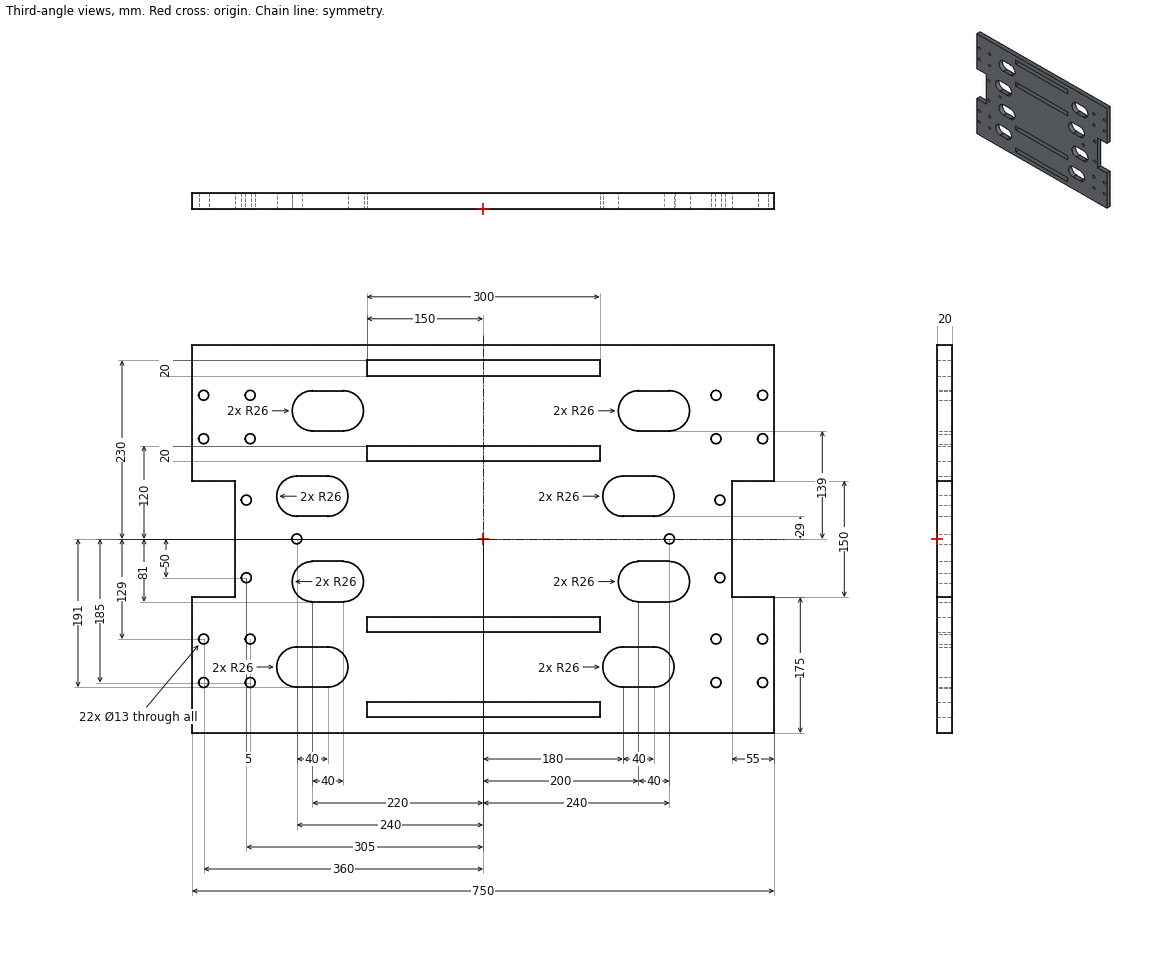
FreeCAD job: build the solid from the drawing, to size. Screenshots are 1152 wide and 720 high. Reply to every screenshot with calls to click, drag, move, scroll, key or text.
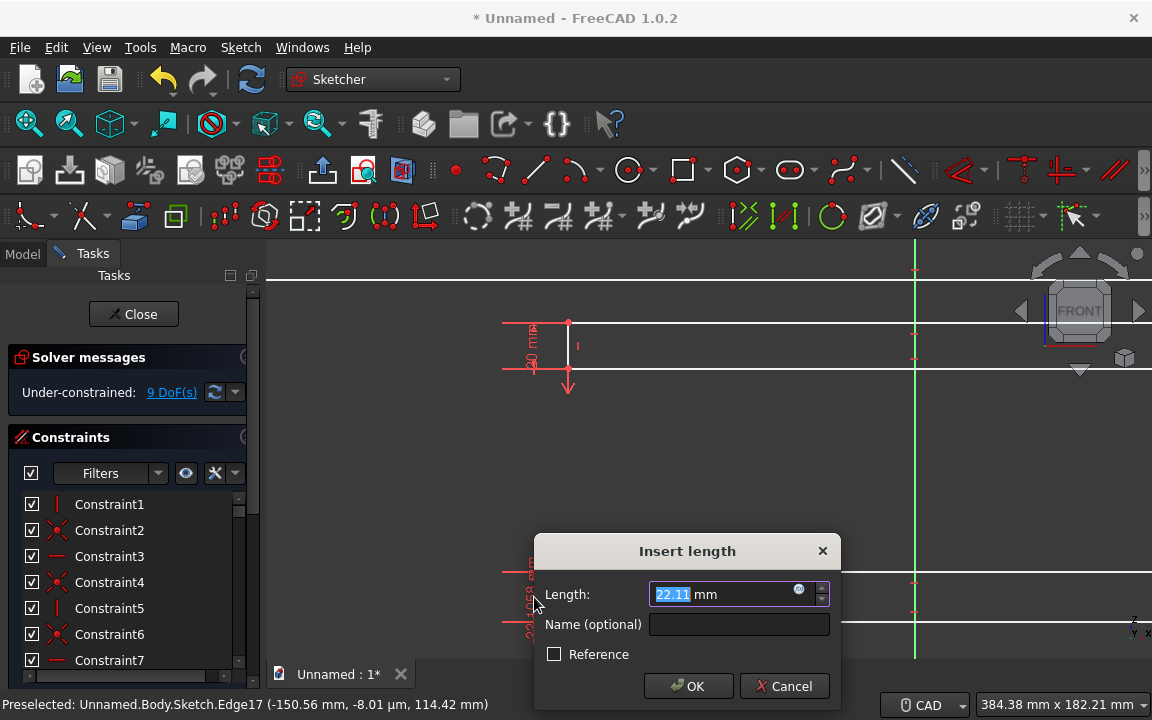
text(20)
key(Return)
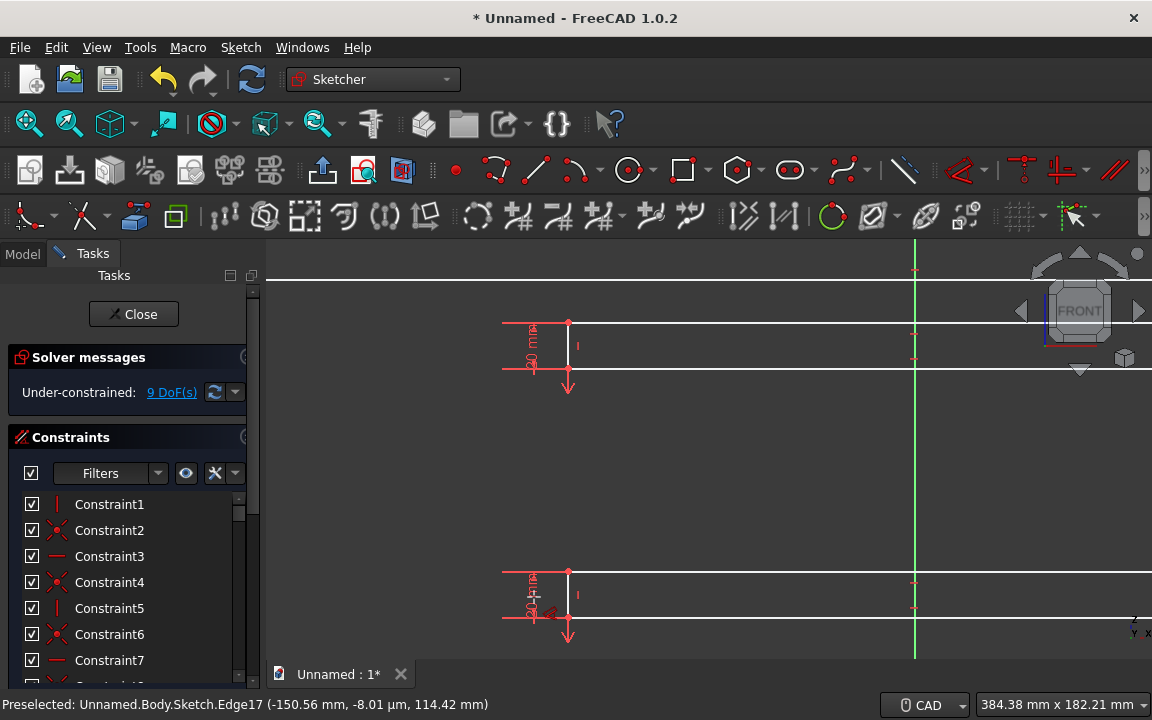
scroll(571, 347, down, 8)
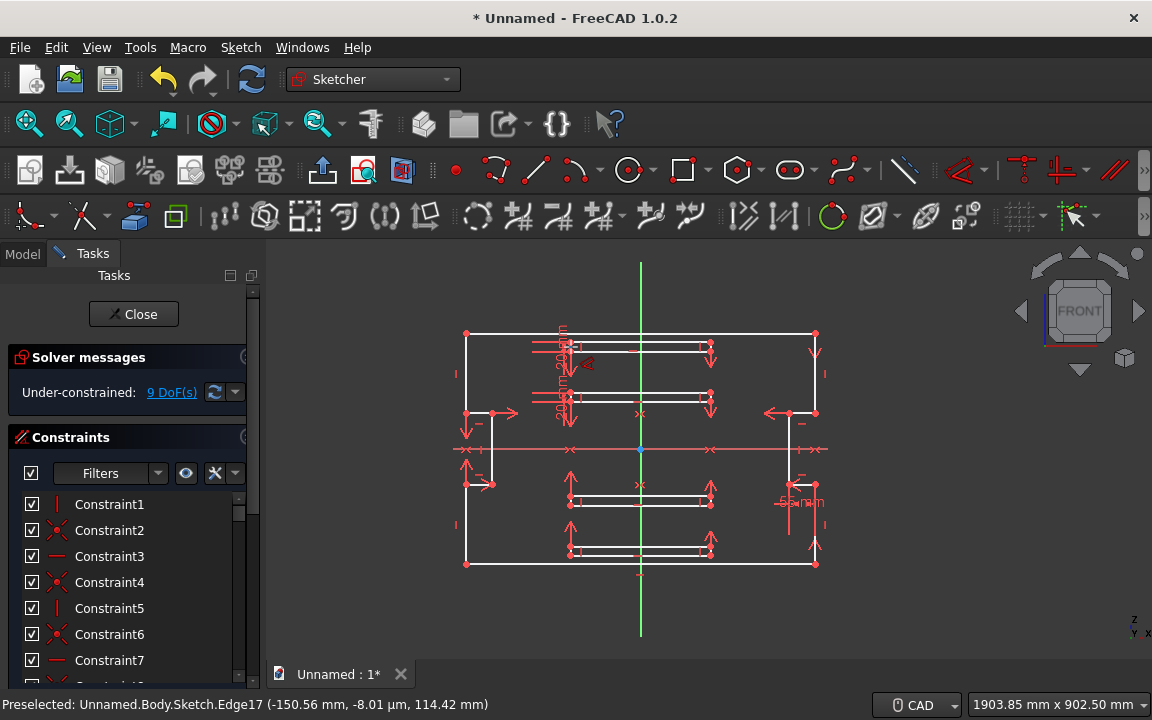
click(789, 435)
click(823, 433)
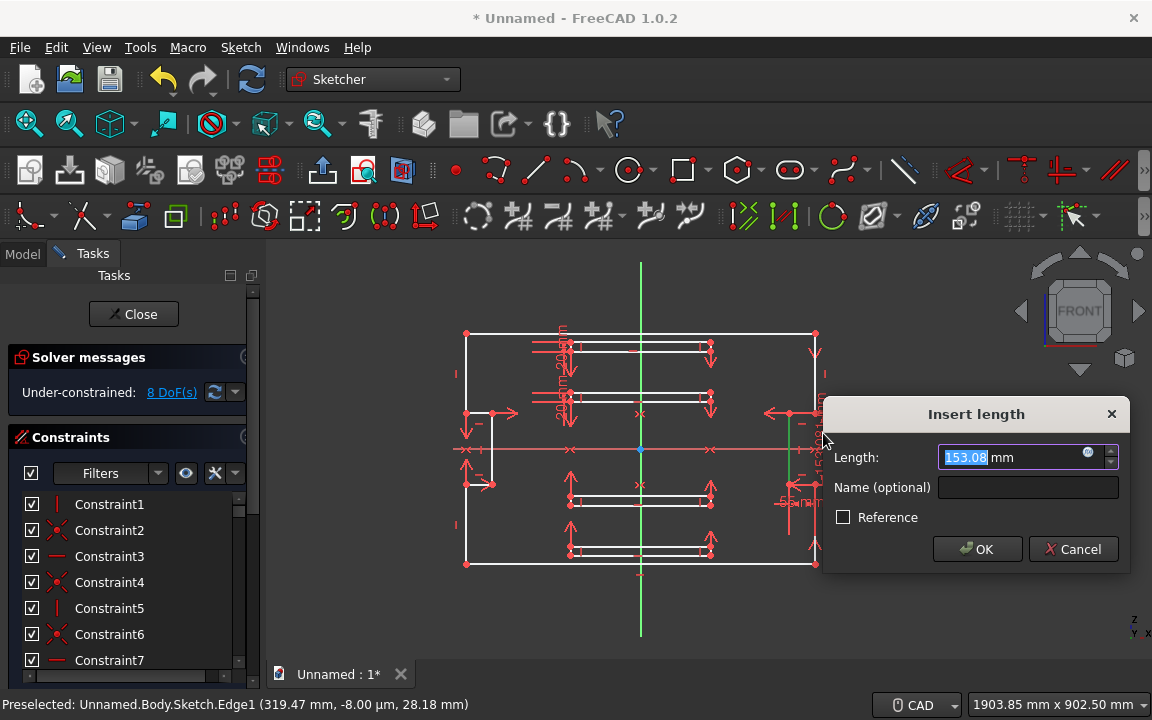
text(150)
key(Return)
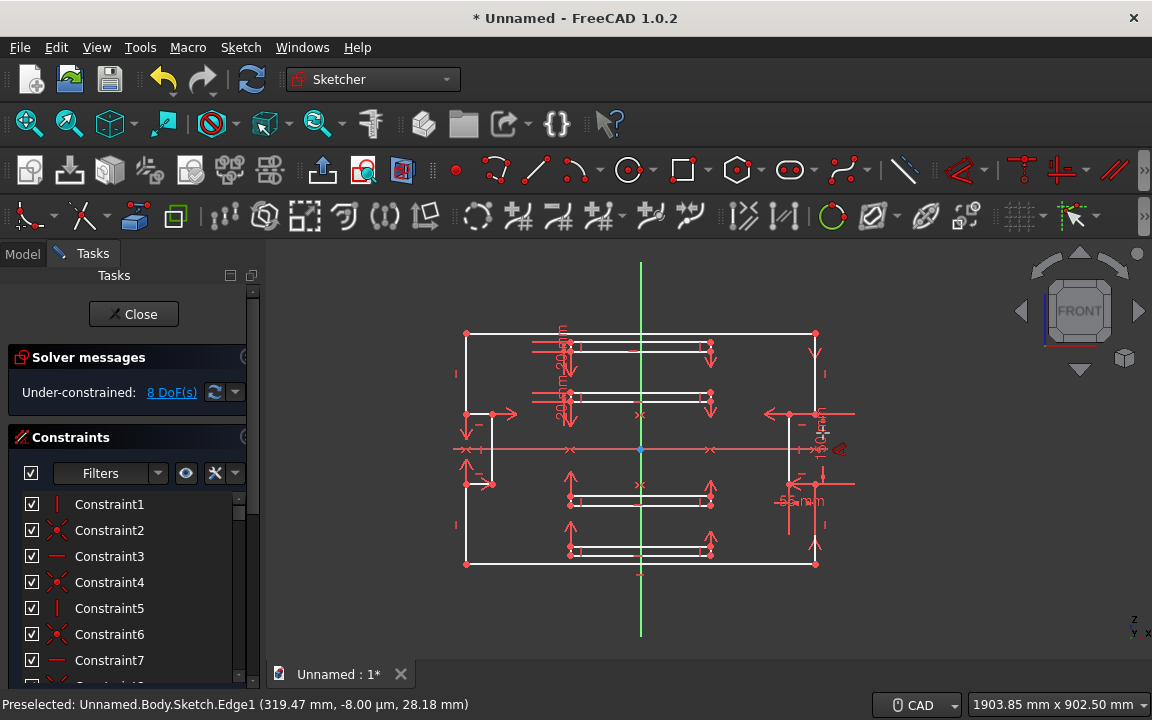
click(815, 508)
click(849, 524)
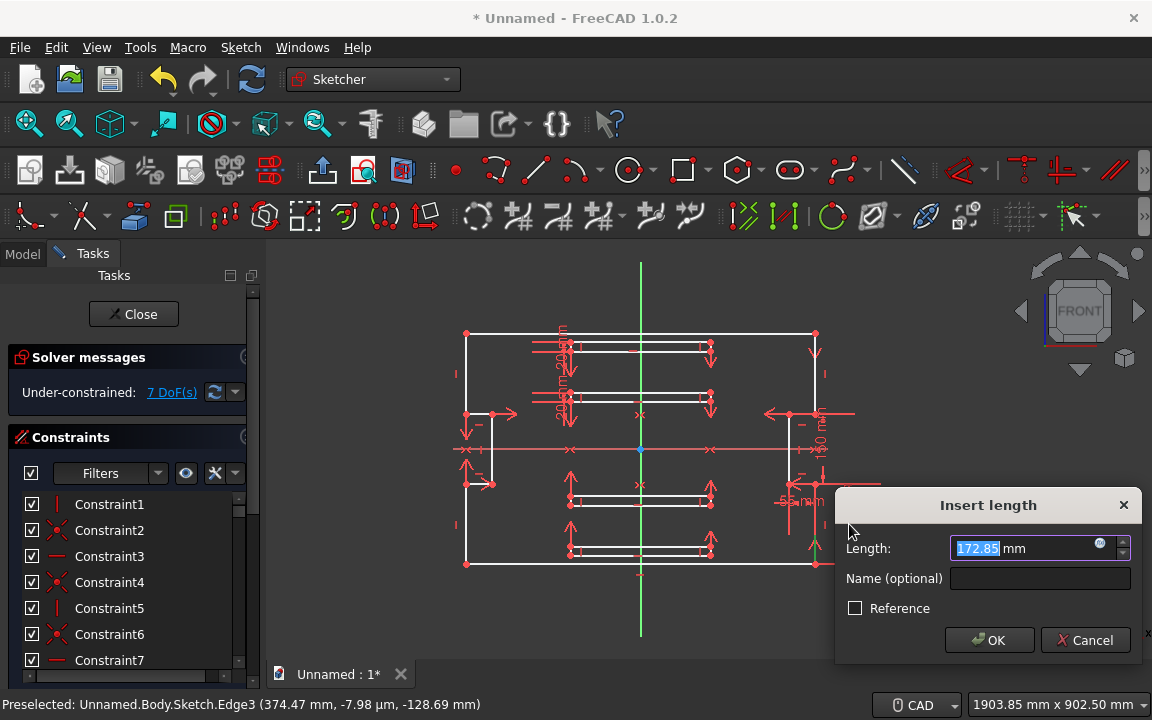
text(175)
key(Return)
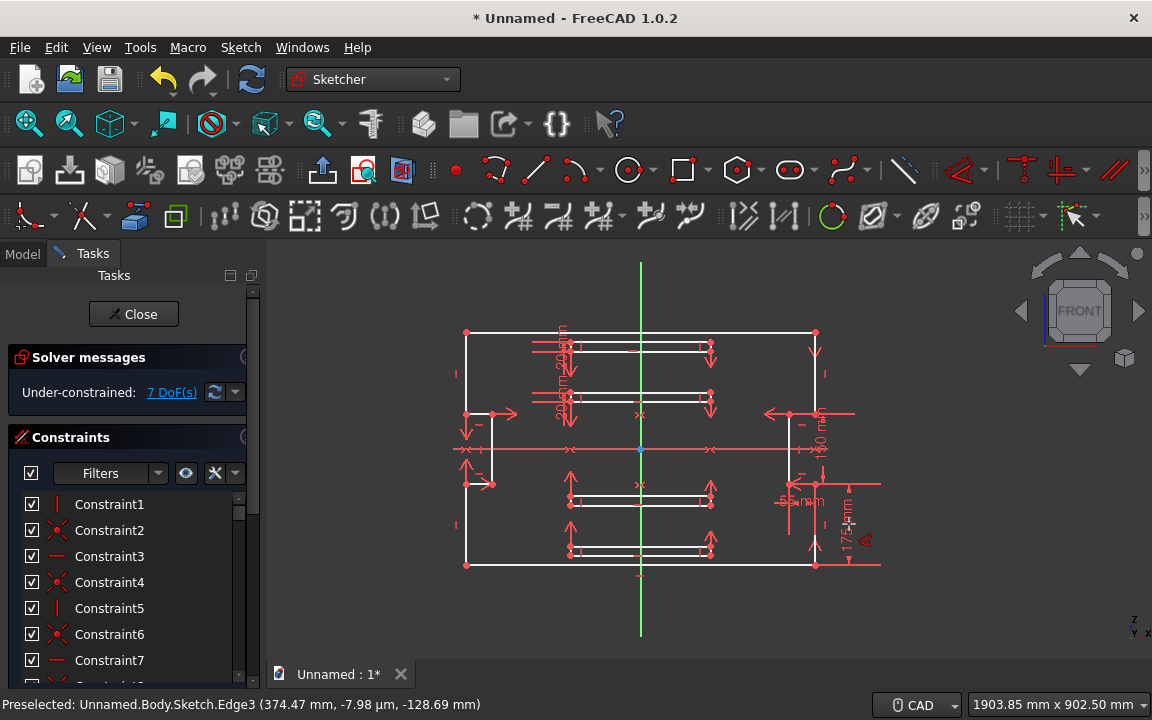
scroll(710, 565, up, 2)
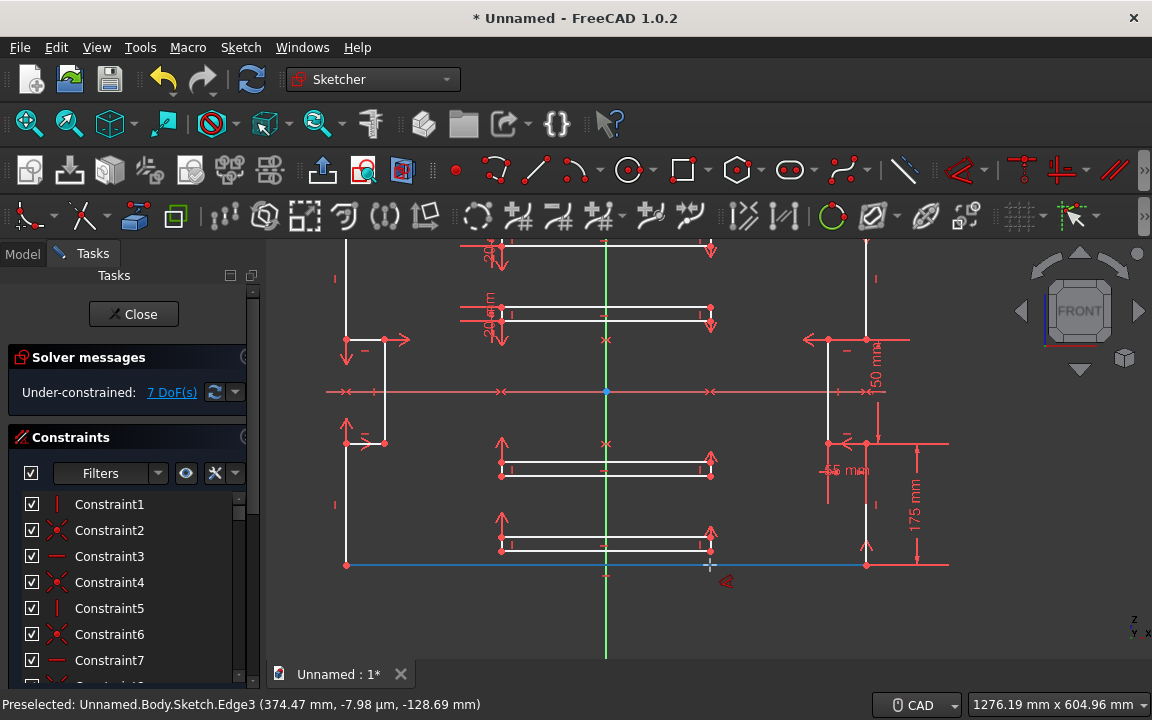
click(710, 565)
click(487, 599)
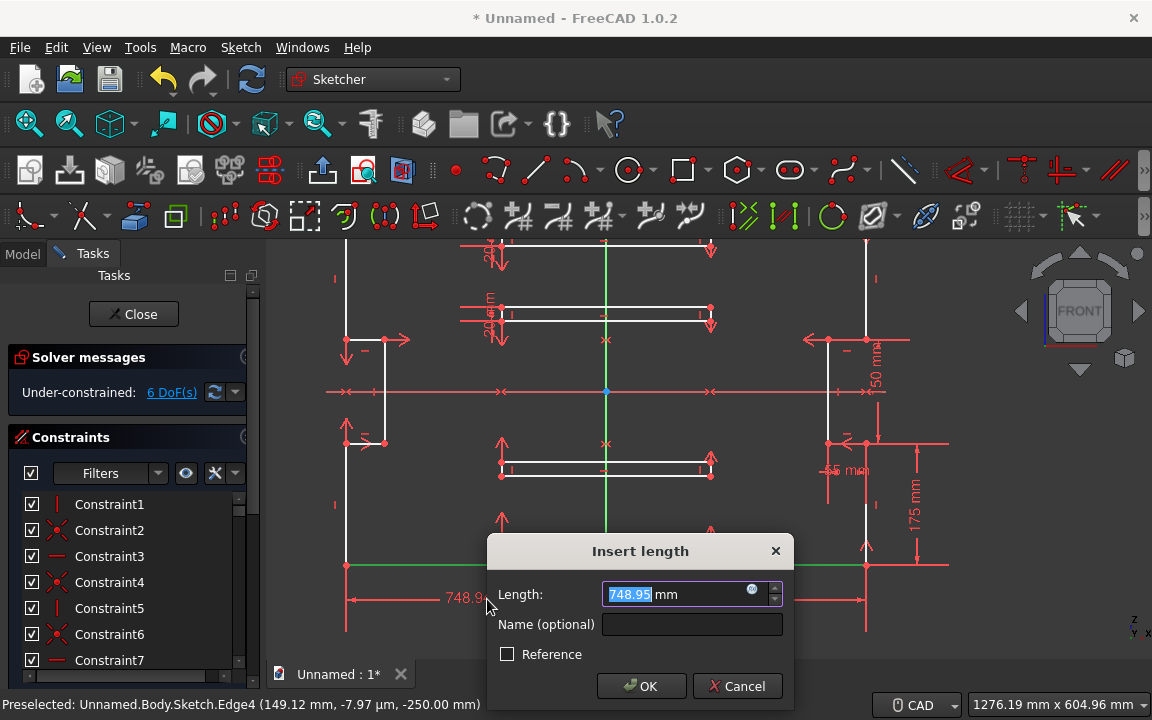
text(750)
key(Return)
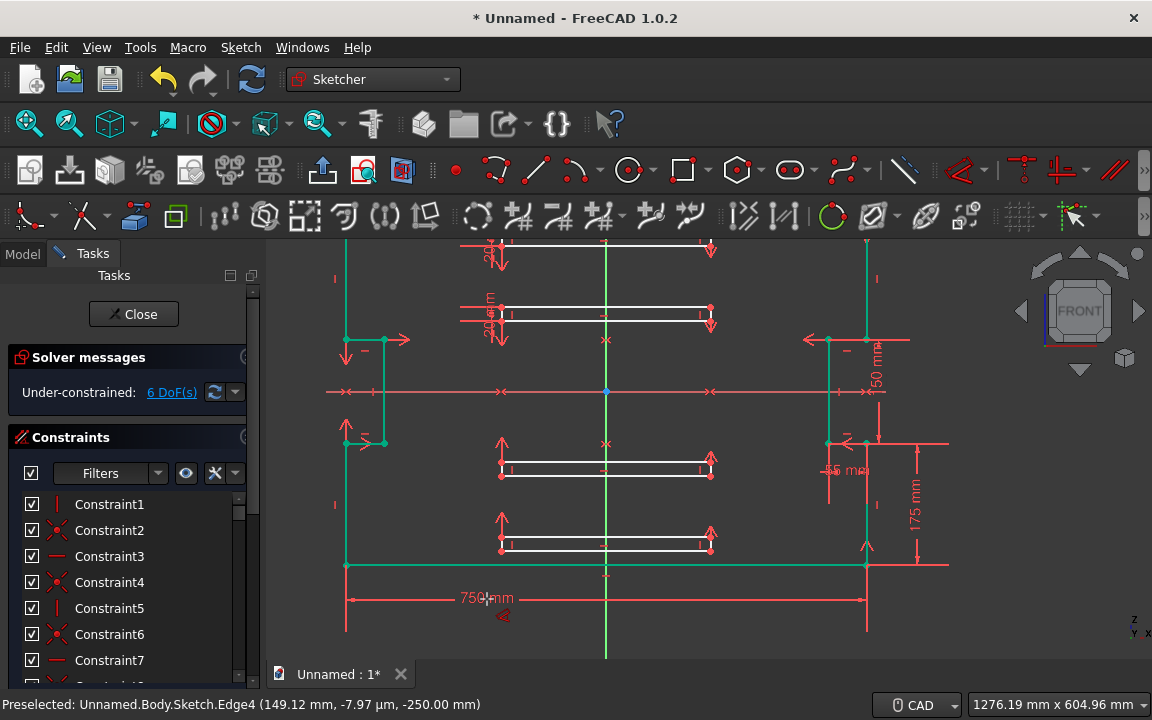
scroll(710, 565, down, 2)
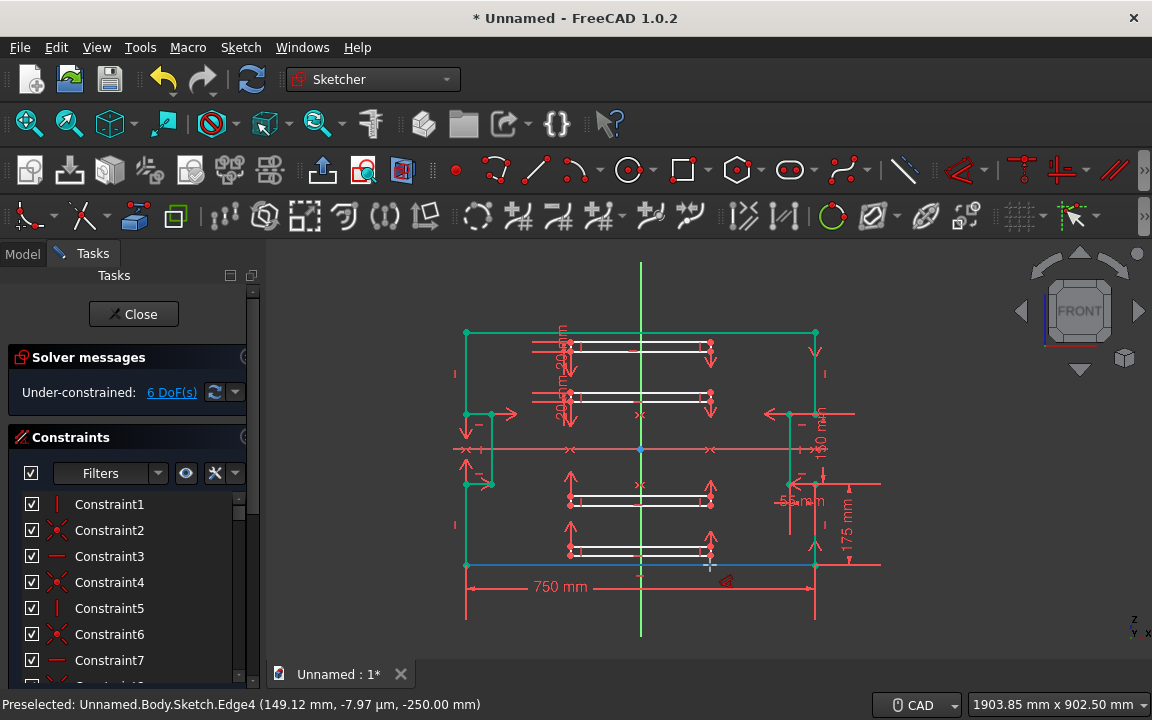
scroll(613, 352, up, 2)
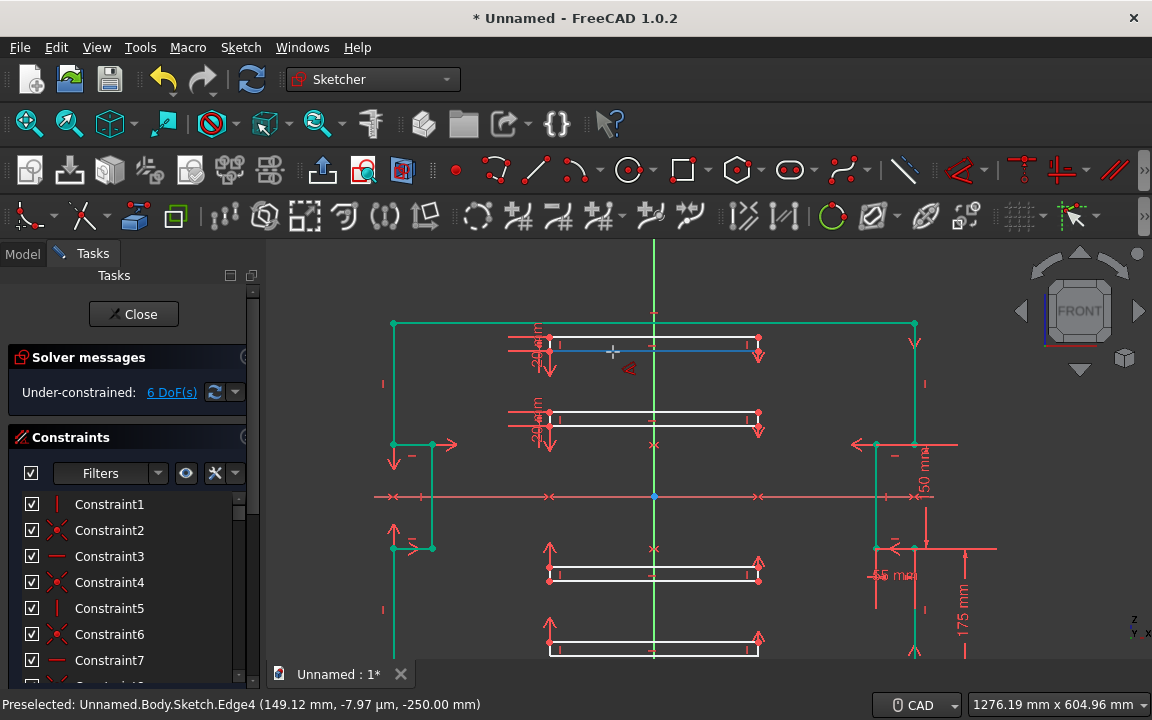
click(612, 351)
click(606, 385)